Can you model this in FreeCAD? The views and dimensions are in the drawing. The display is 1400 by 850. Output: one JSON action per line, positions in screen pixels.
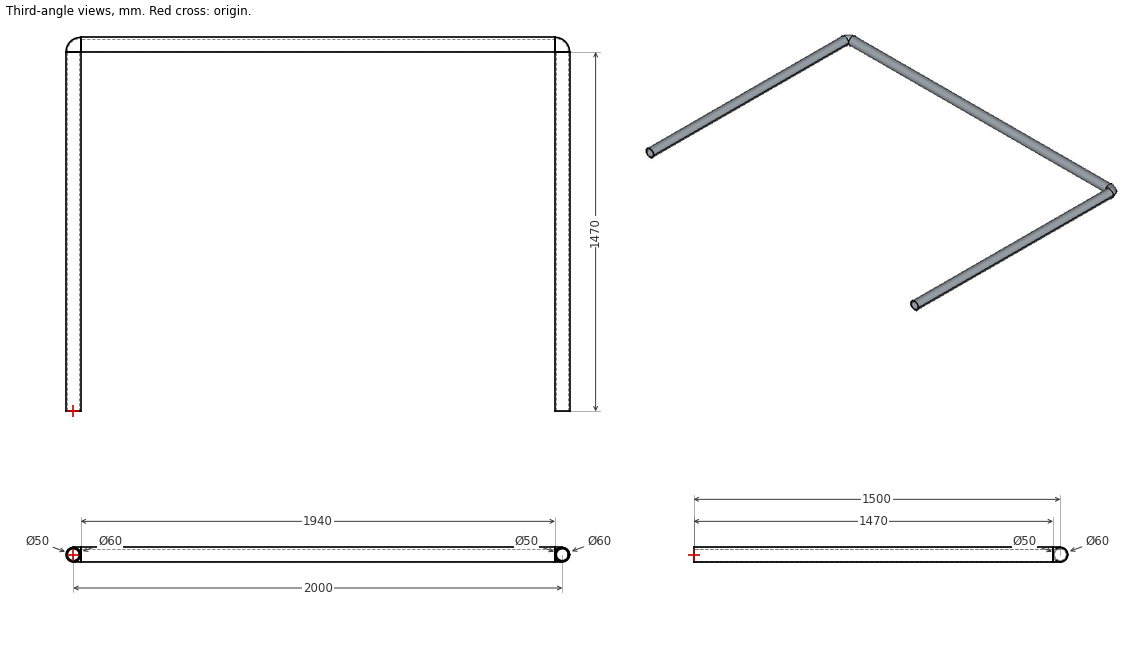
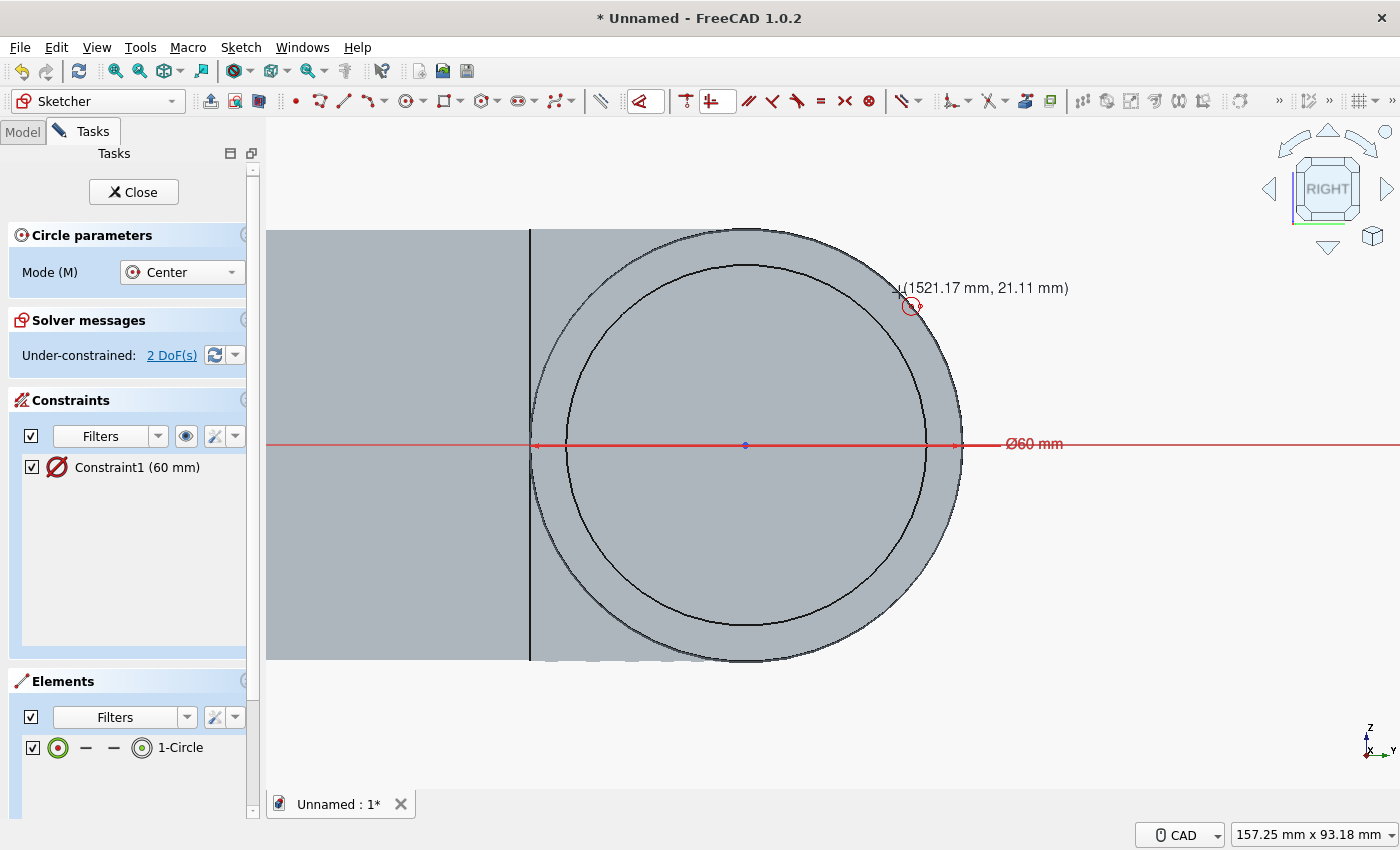
{"action": "left_click", "coordinate": [746, 446]}
{"action": "mouse_move", "coordinate": [874, 318]}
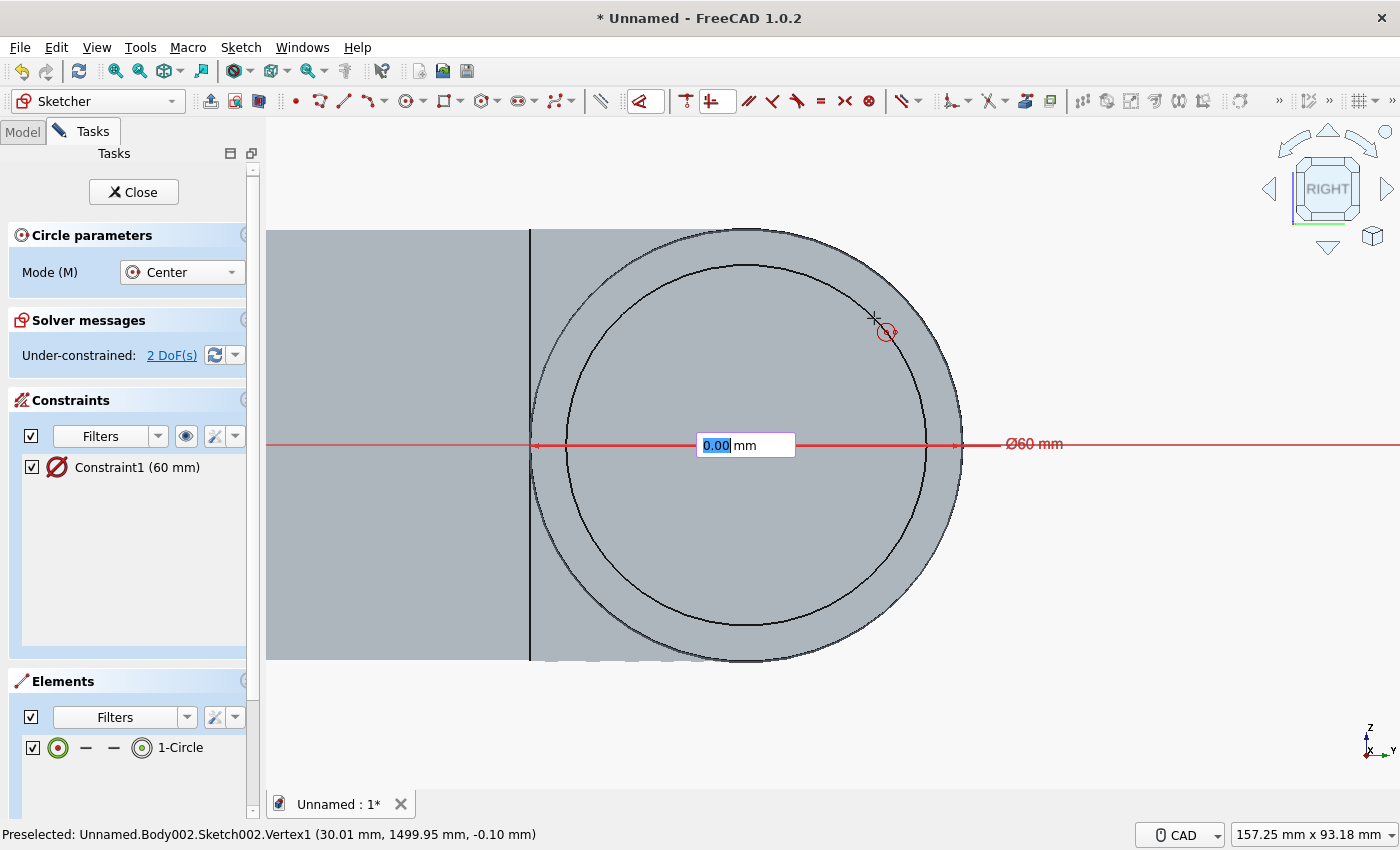
{"action": "type", "text": "50"}
{"action": "key", "text": "Return"}
{"action": "key", "text": "Escape"}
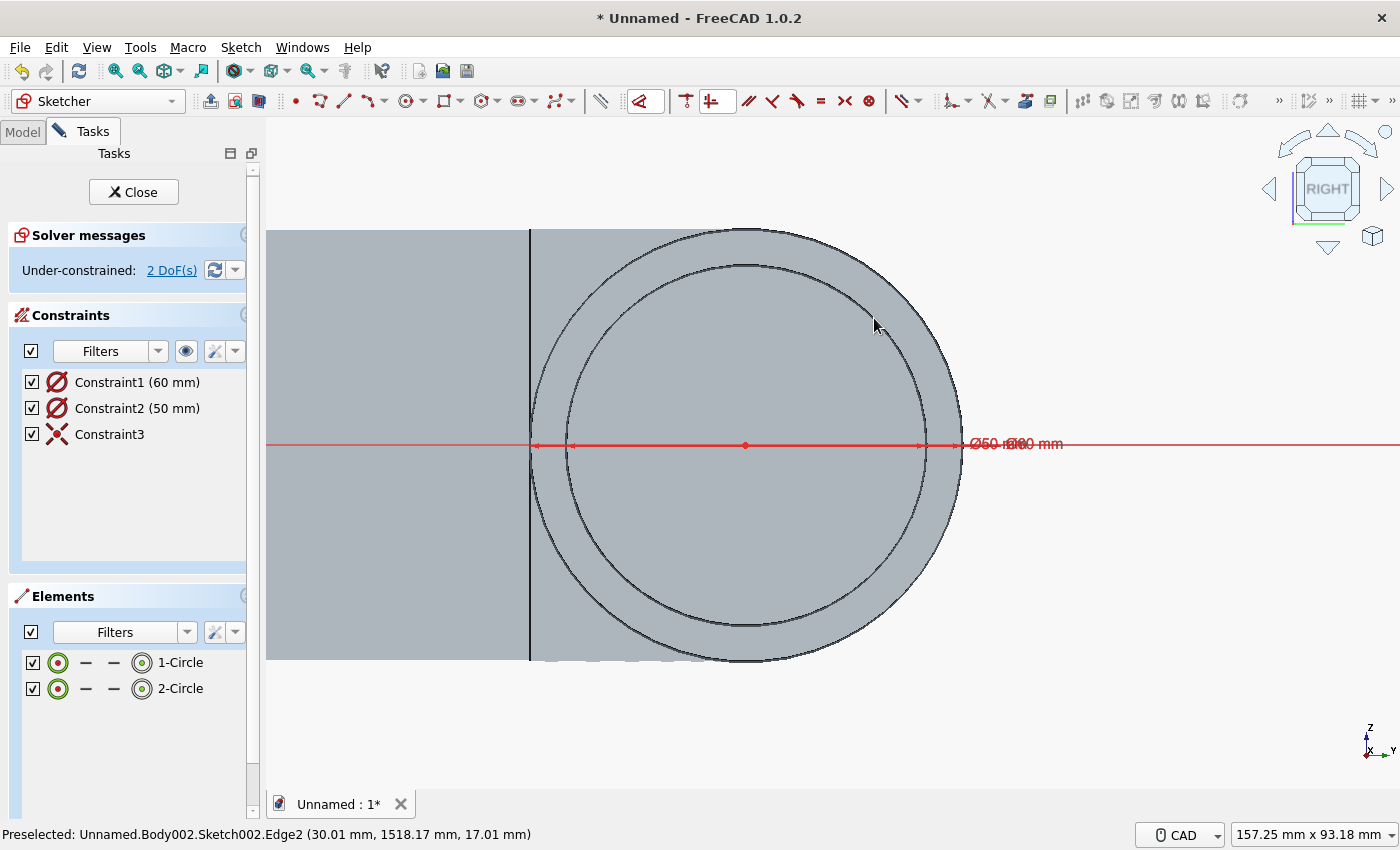
{"action": "left_click", "coordinate": [746, 446]}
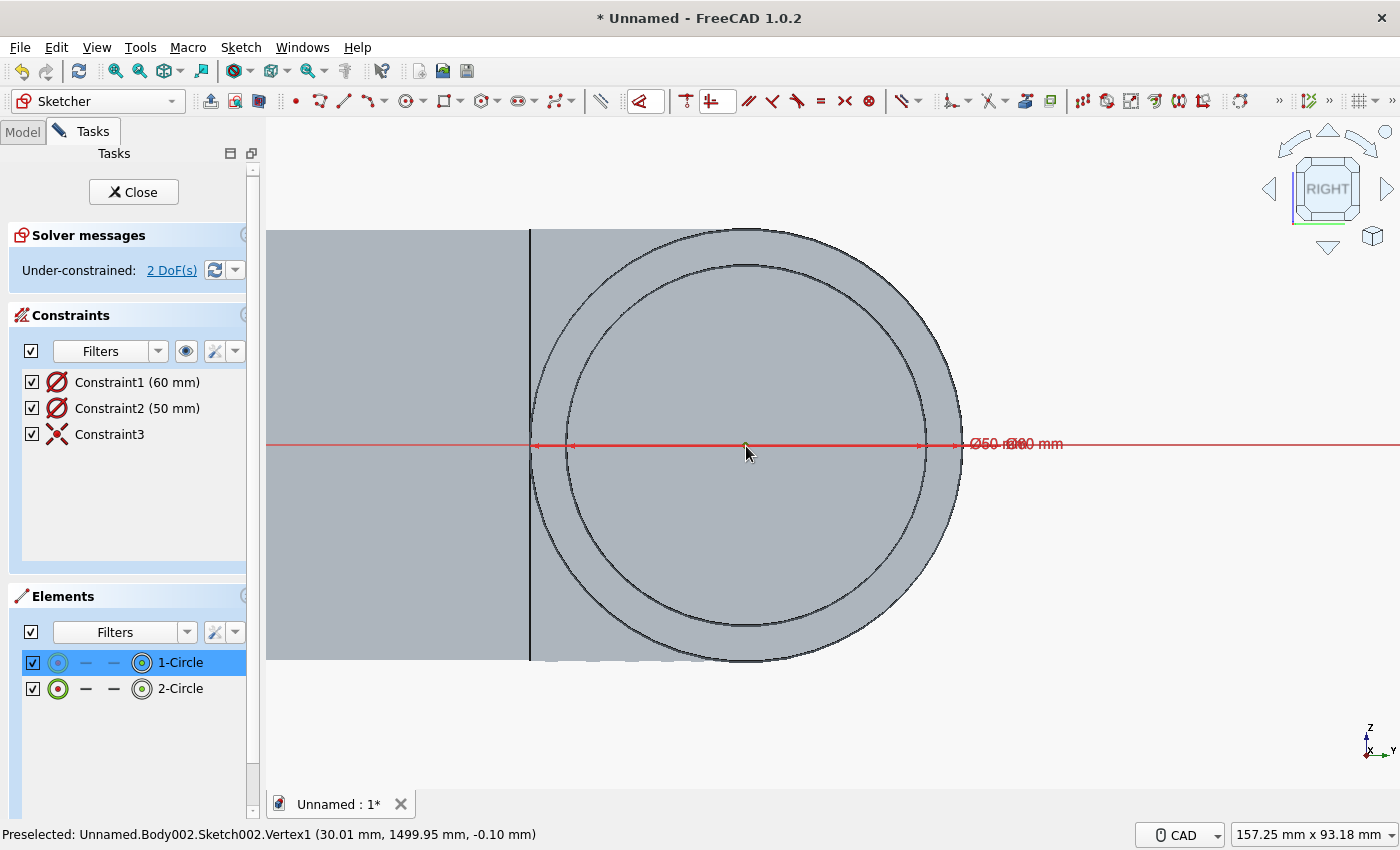
{"action": "left_click", "coordinate": [361, 445]}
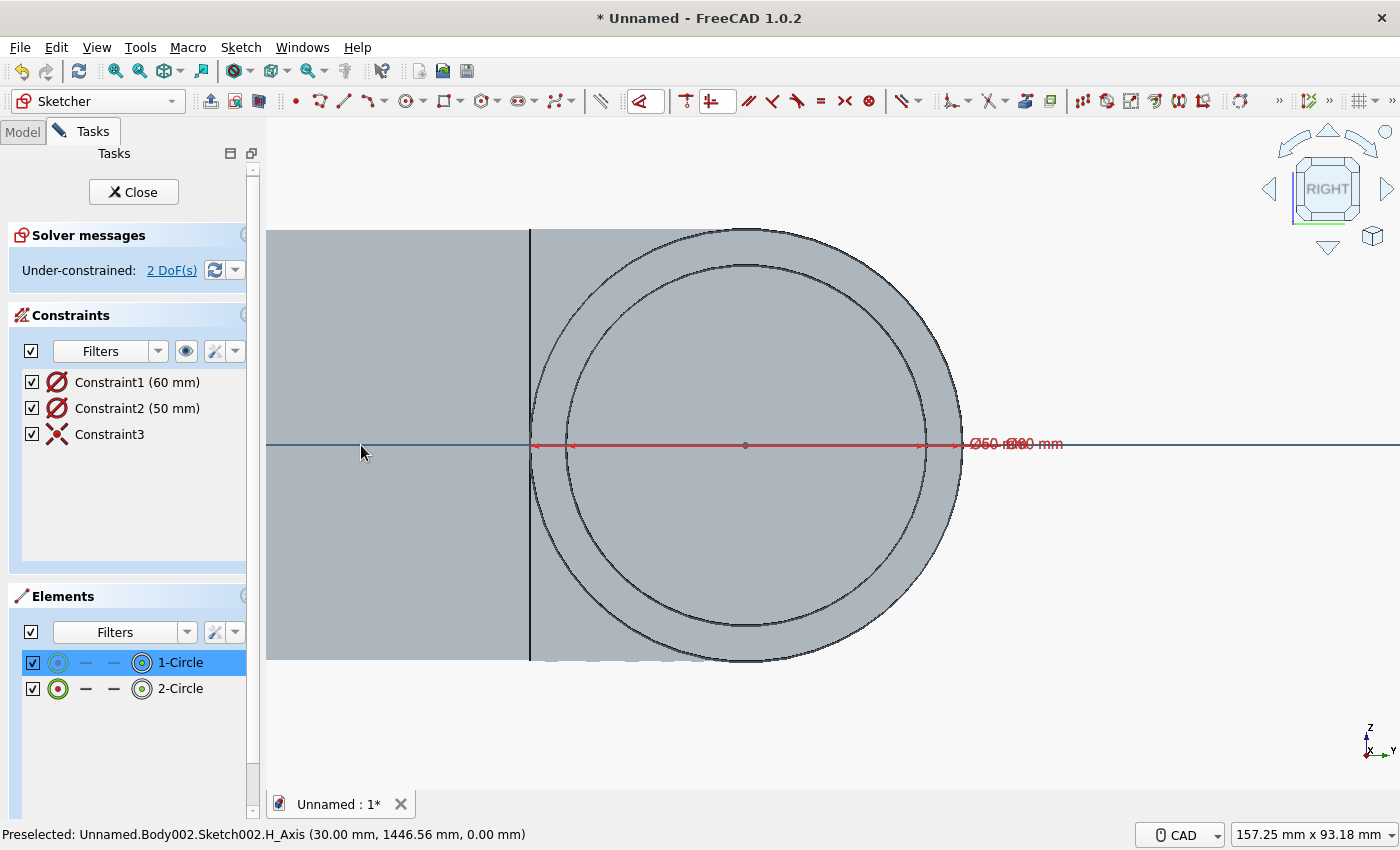
{"action": "left_click", "coordinate": [686, 102]}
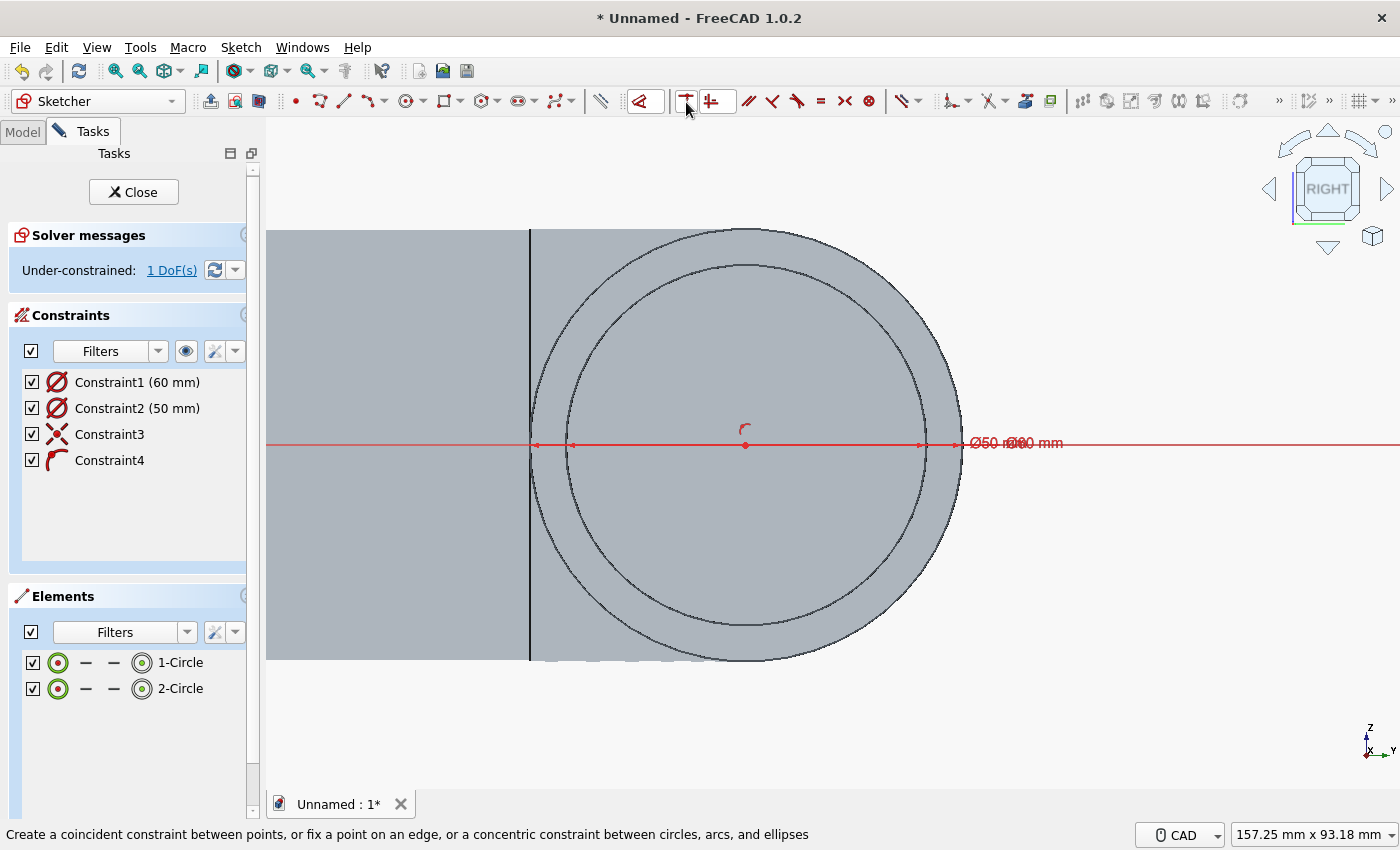
{"action": "left_click", "coordinate": [640, 102]}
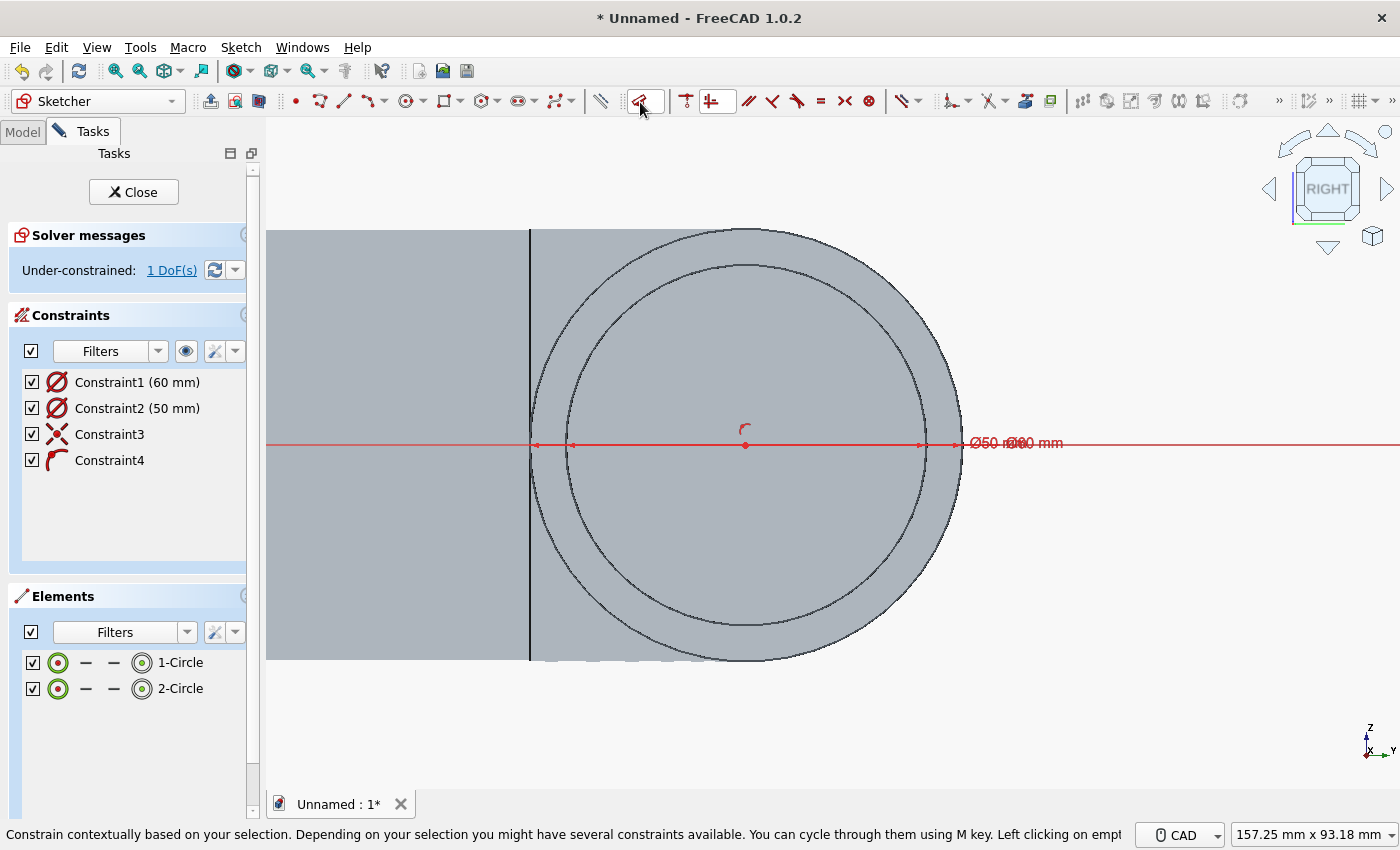
{"action": "left_click", "coordinate": [746, 445]}
{"action": "left_click", "coordinate": [416, 479]}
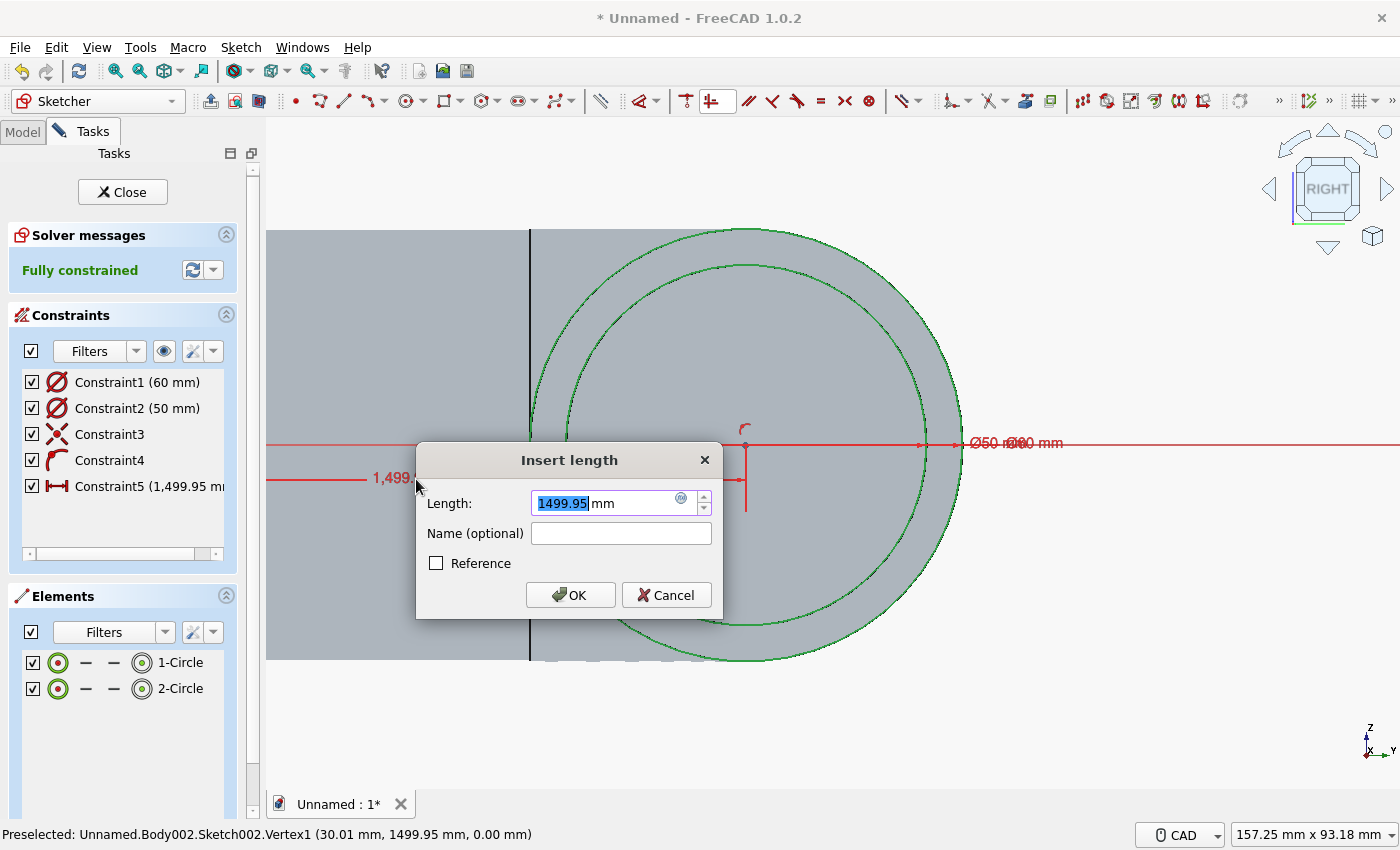
{"action": "type", "text": "1500"}
{"action": "key", "text": "Return"}
{"action": "key", "text": "Escape"}